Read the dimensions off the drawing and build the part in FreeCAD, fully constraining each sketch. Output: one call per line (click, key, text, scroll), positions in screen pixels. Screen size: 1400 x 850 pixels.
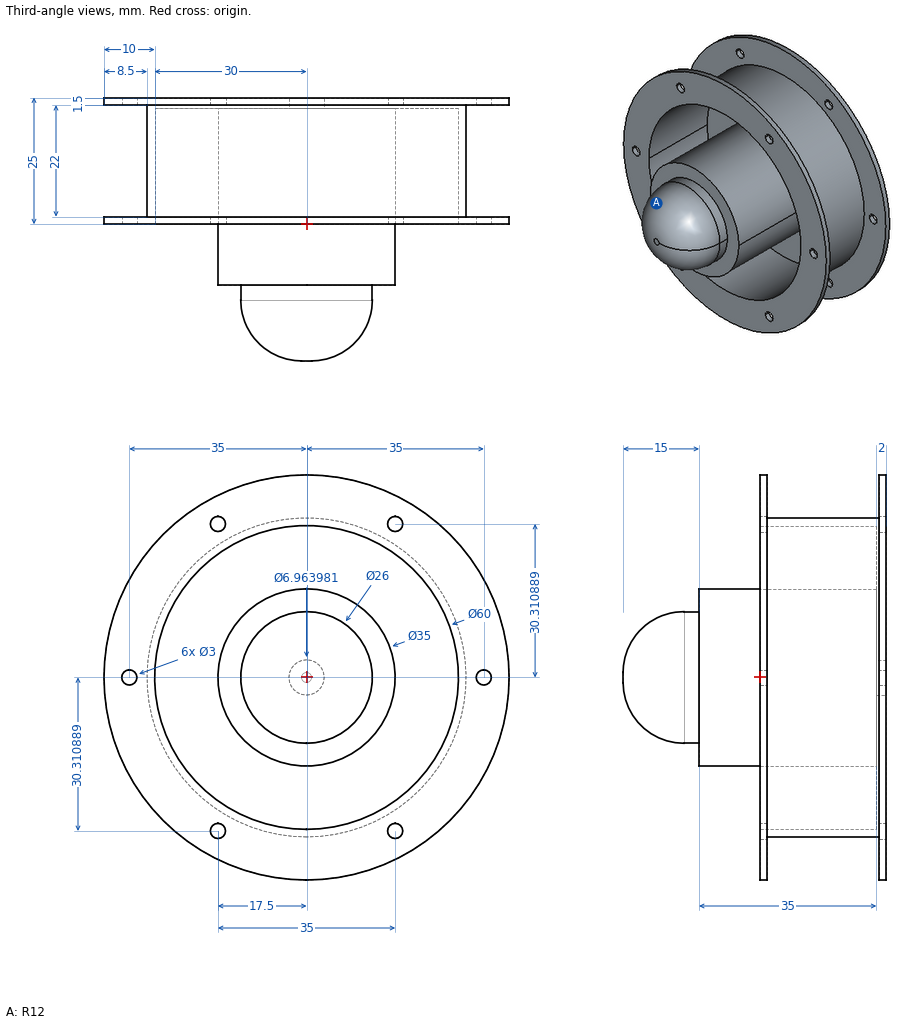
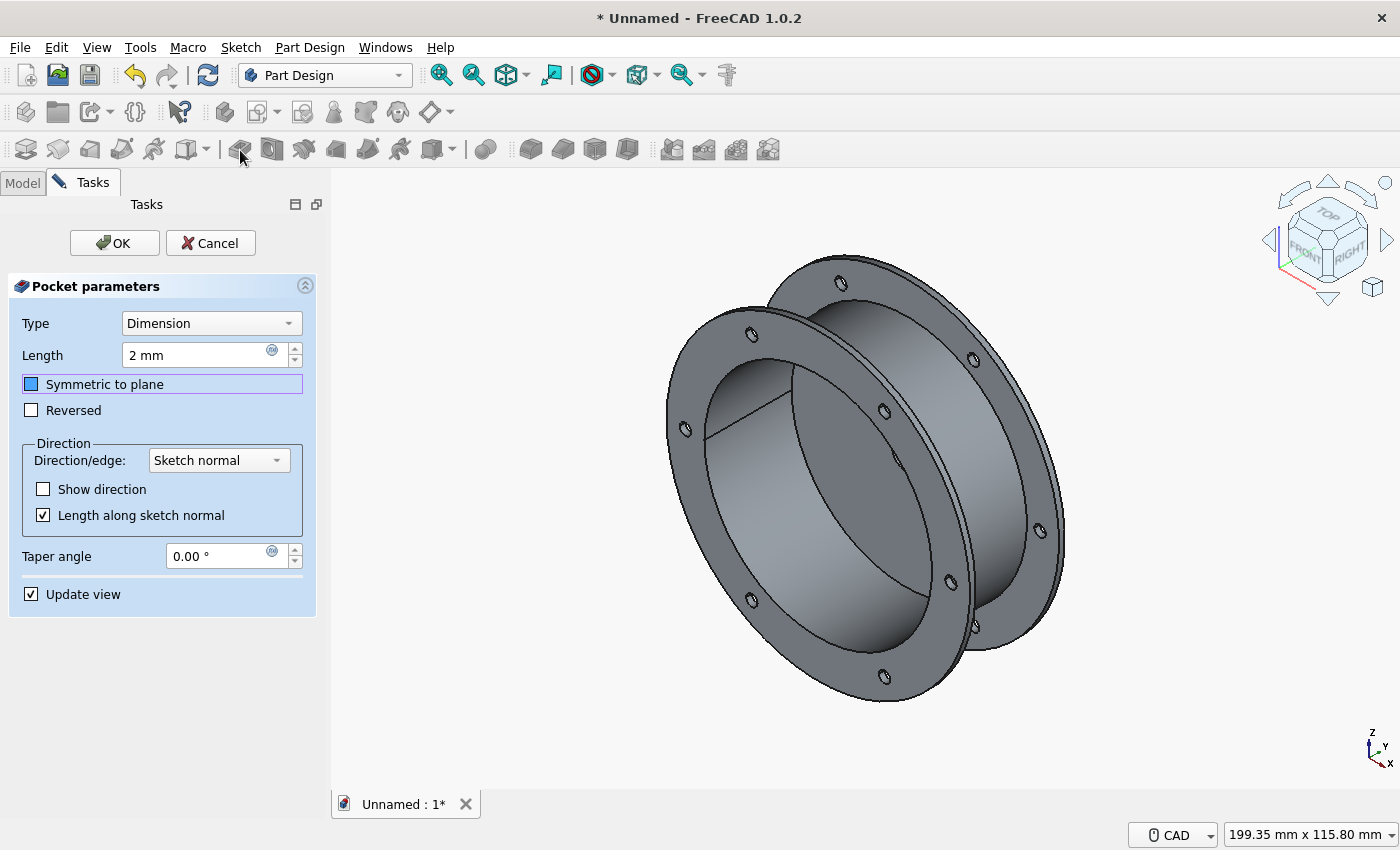
click(115, 243)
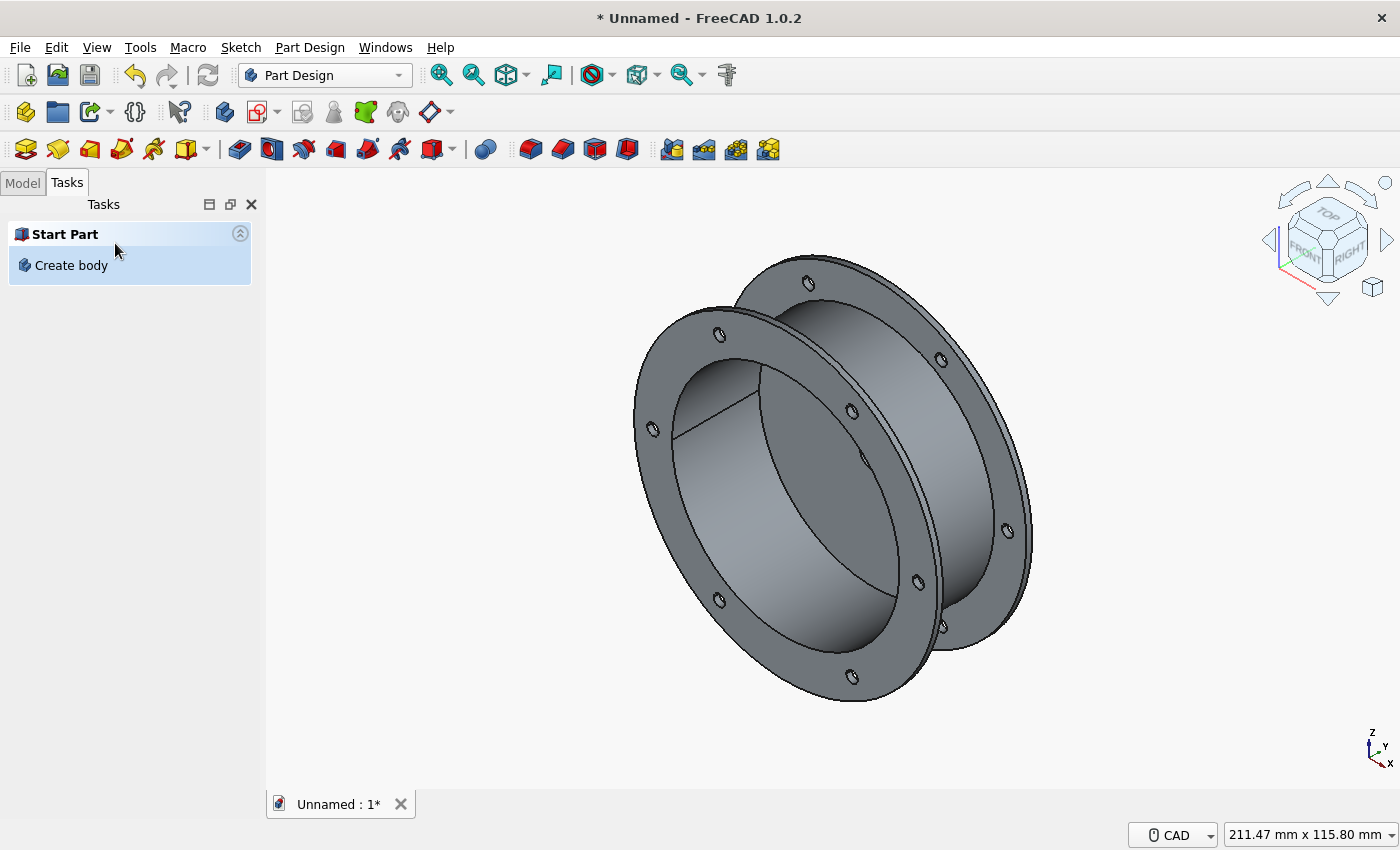
click(873, 530)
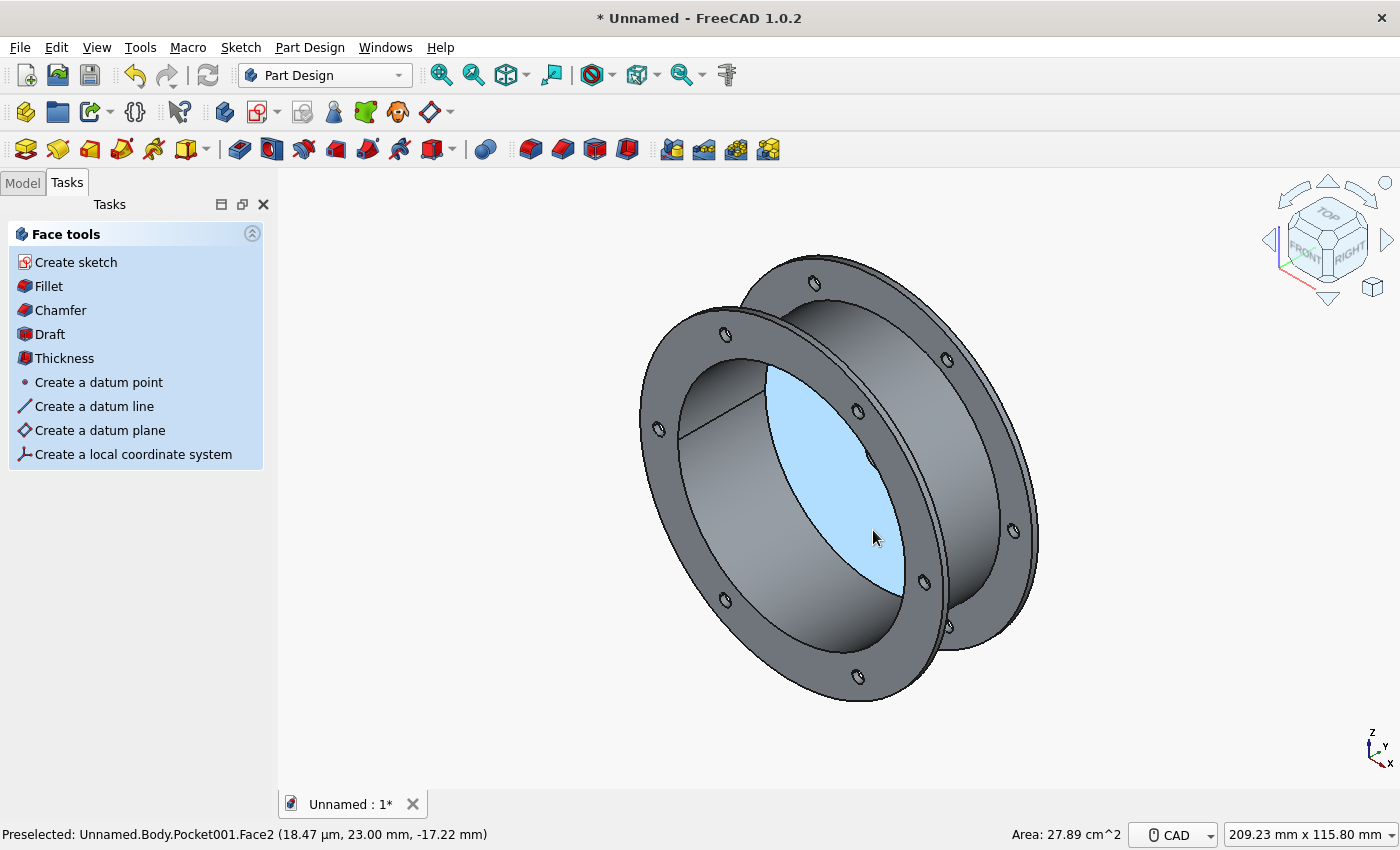
click(258, 112)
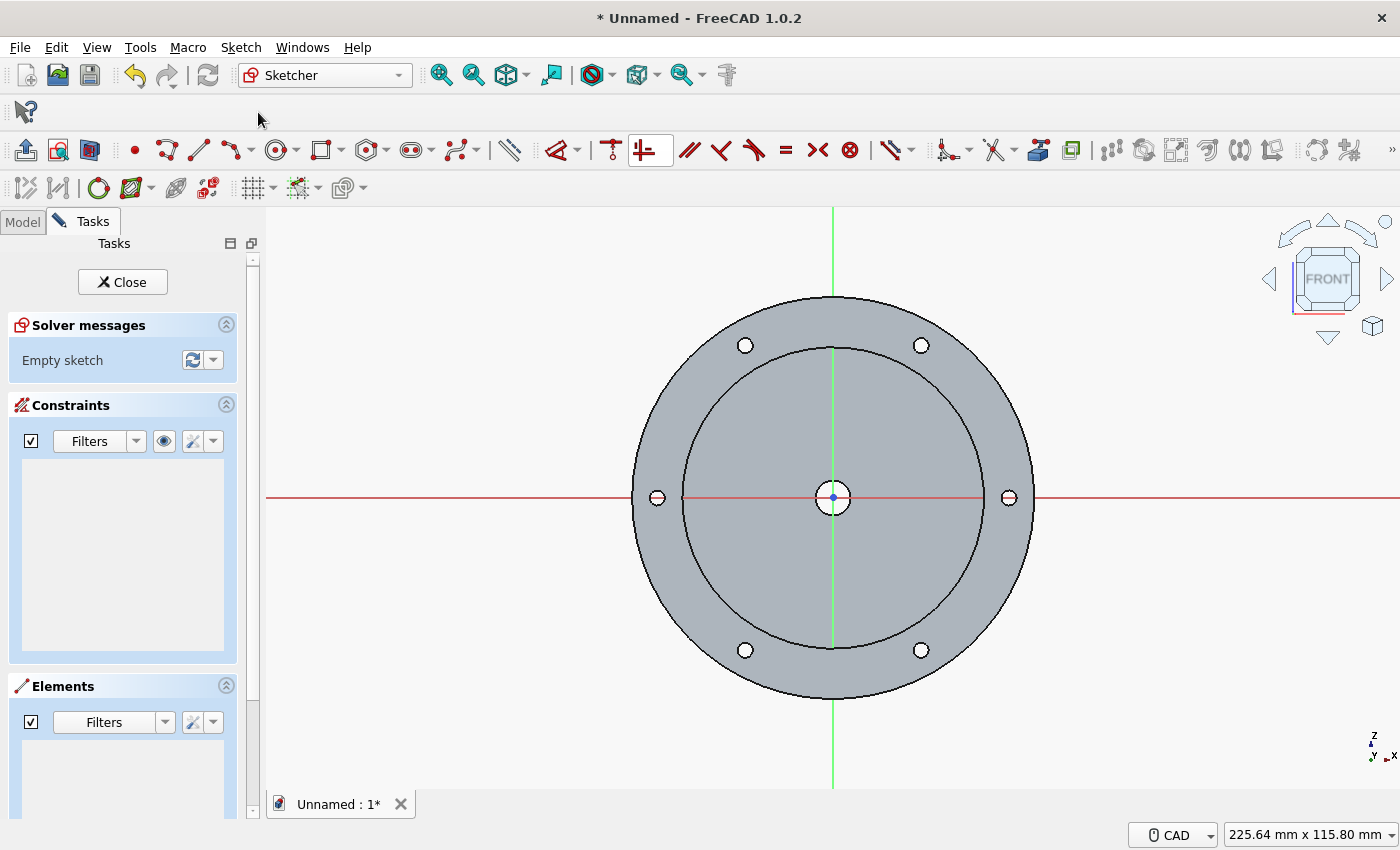
click(90, 150)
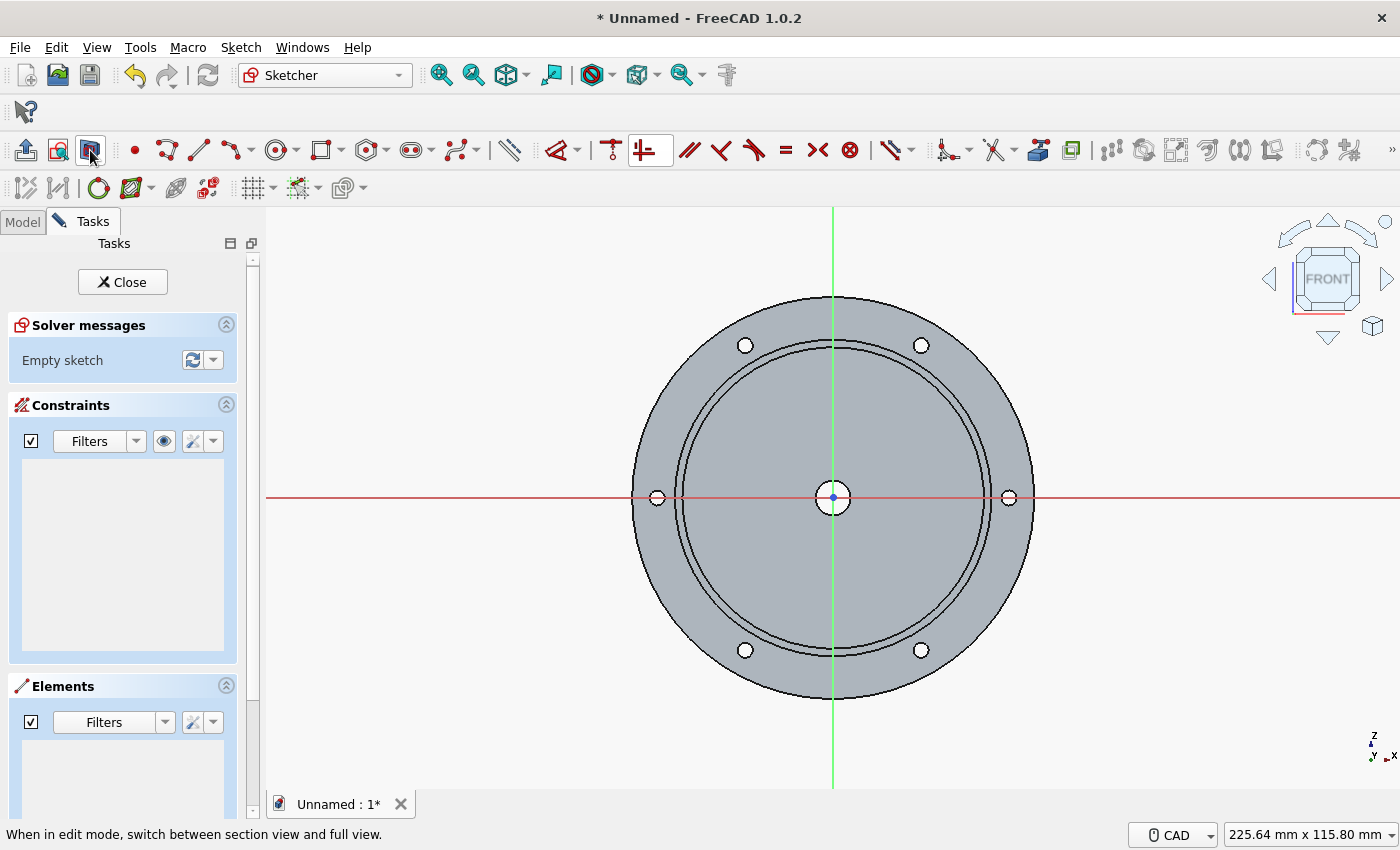
scroll(889, 498, up, 4)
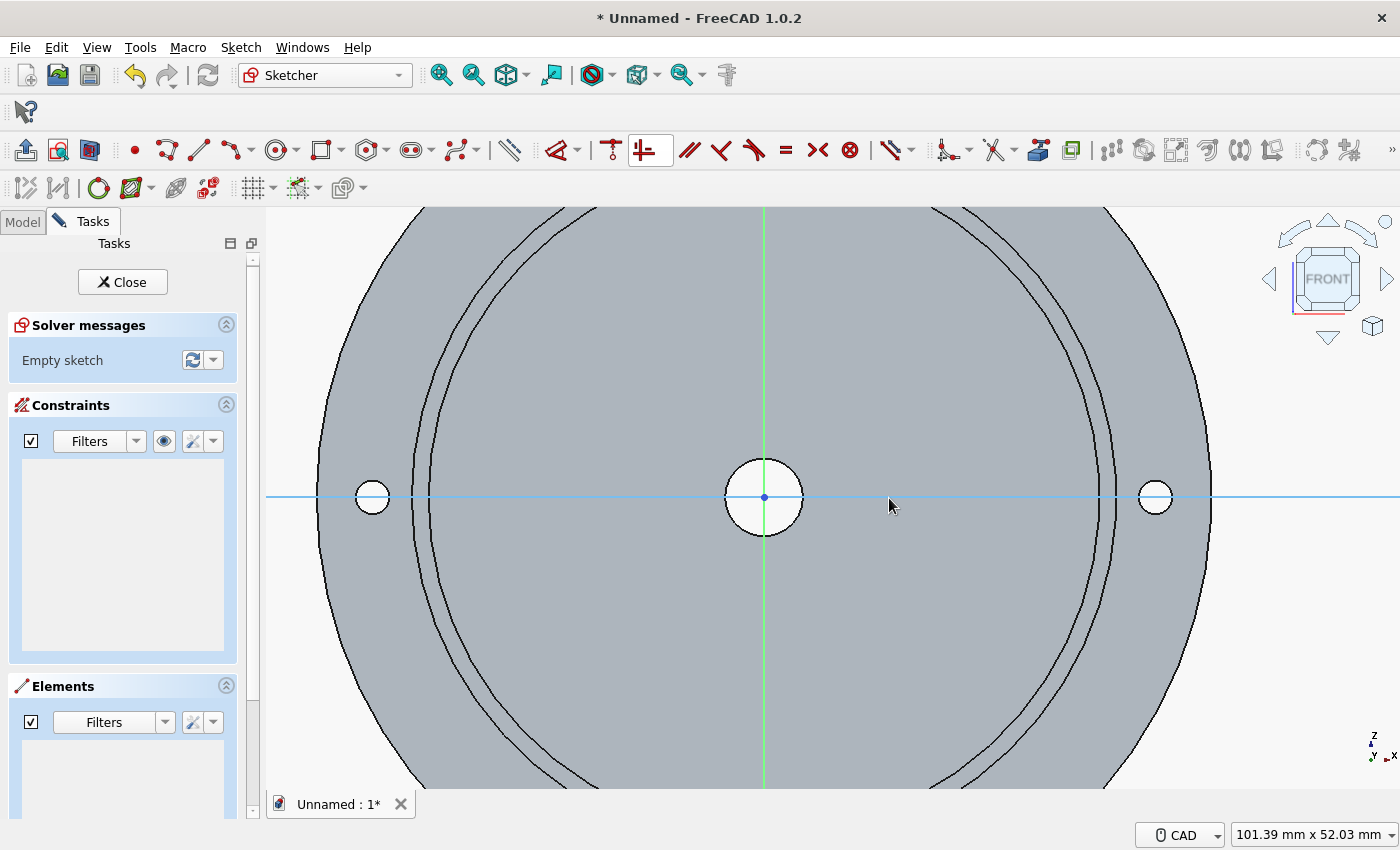
click(276, 150)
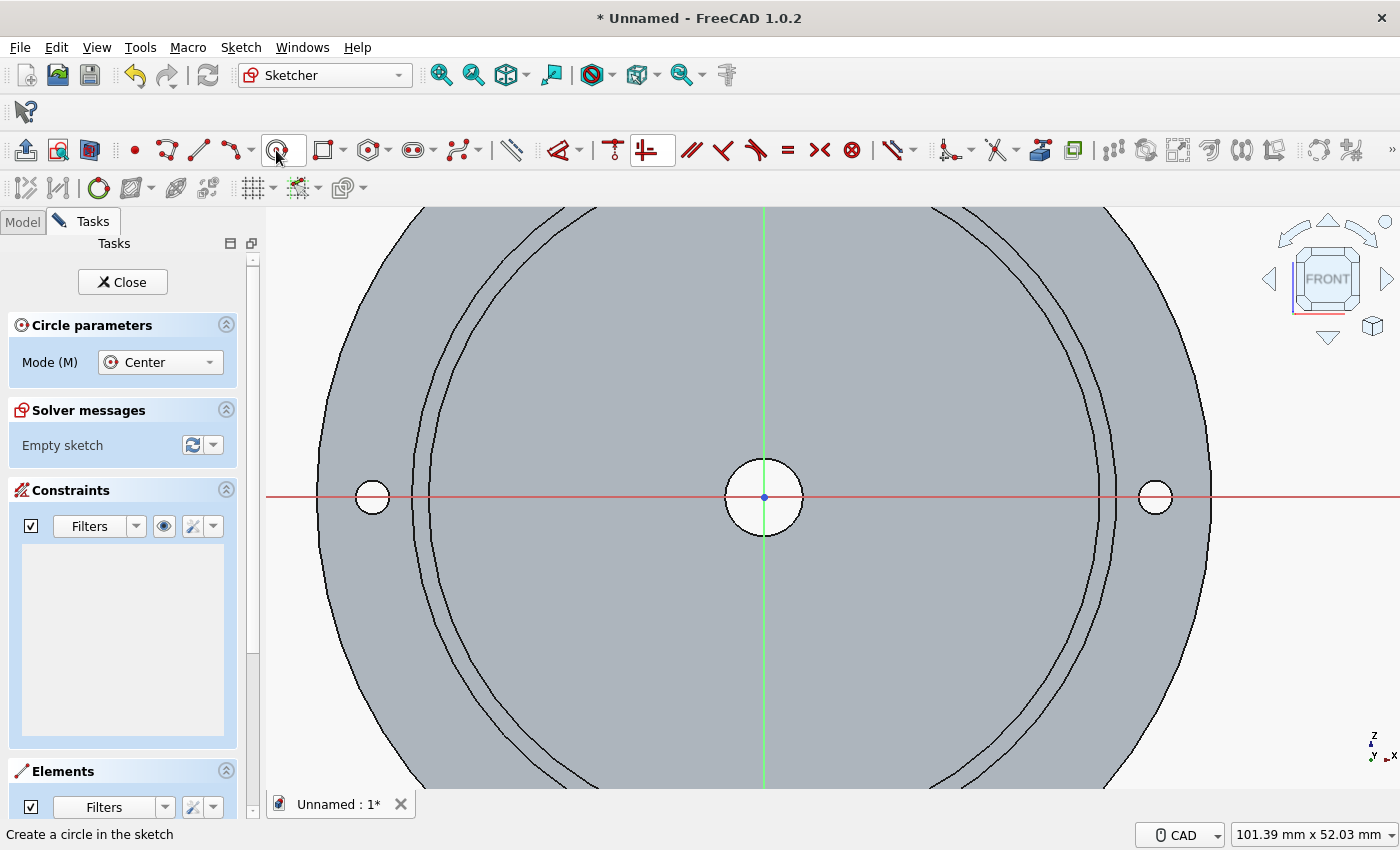
click(764, 497)
click(902, 359)
key(Escape)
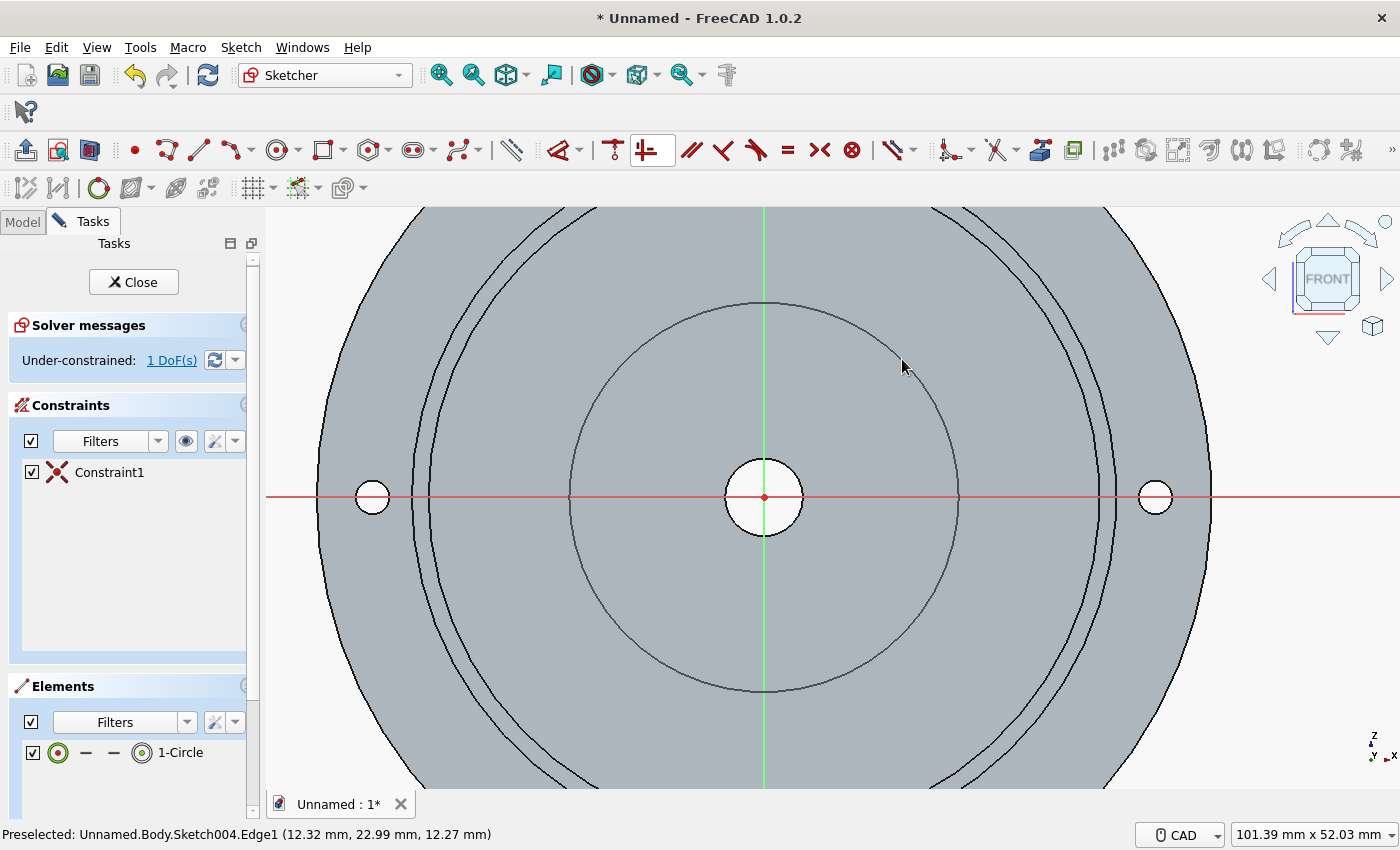
click(558, 150)